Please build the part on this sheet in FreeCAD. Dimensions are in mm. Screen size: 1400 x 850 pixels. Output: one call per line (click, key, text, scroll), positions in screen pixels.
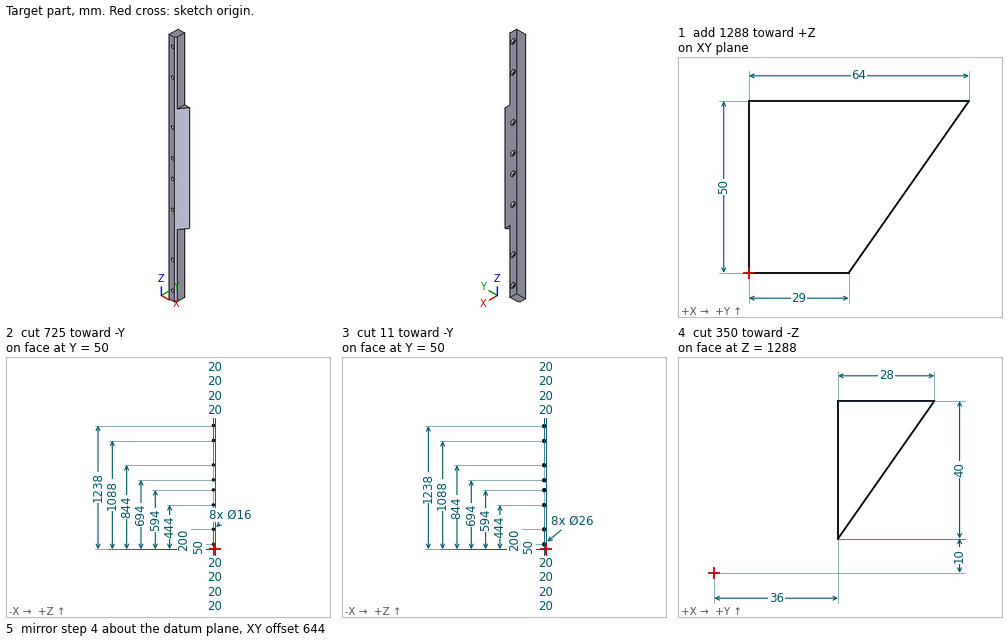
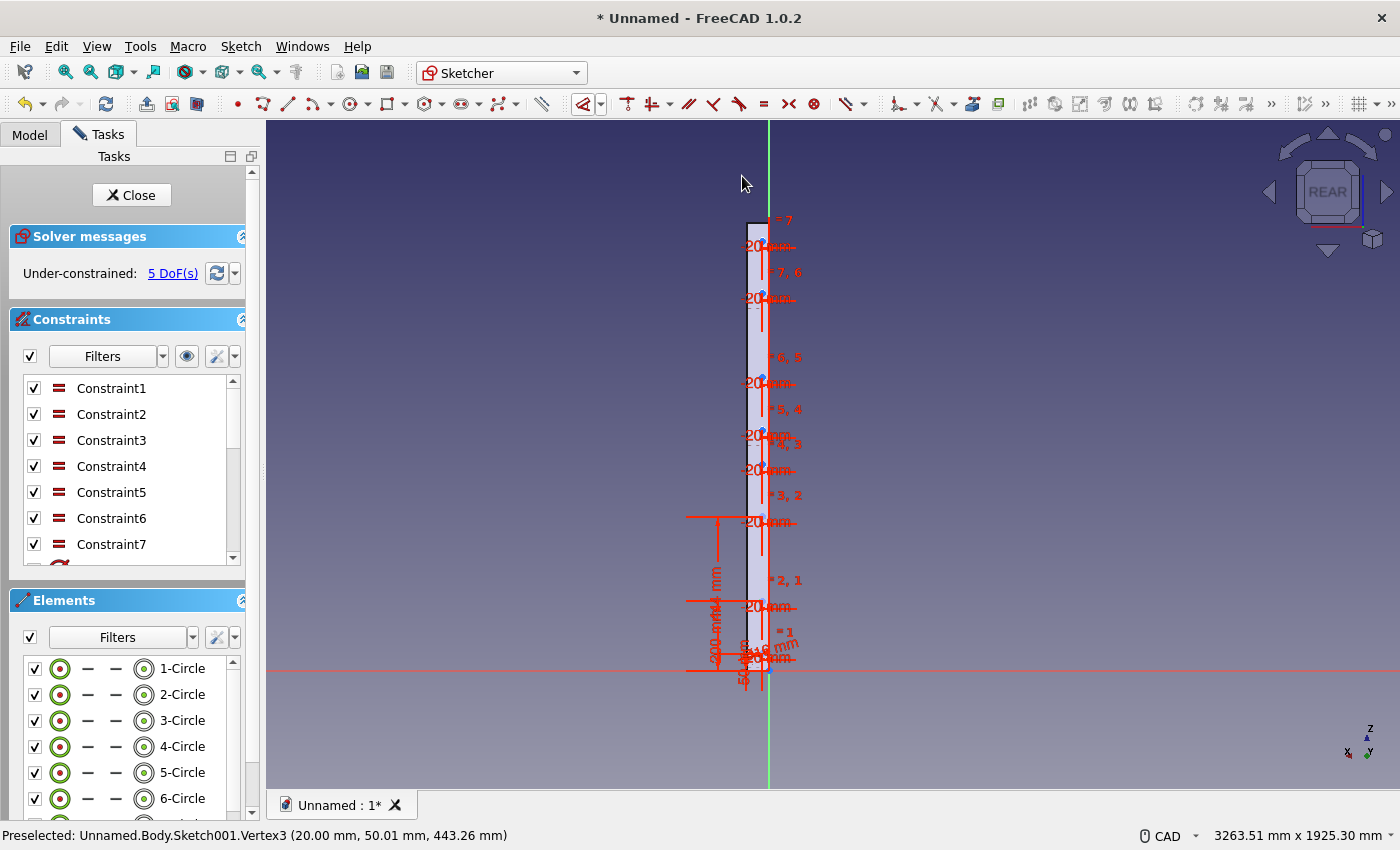
click(762, 465)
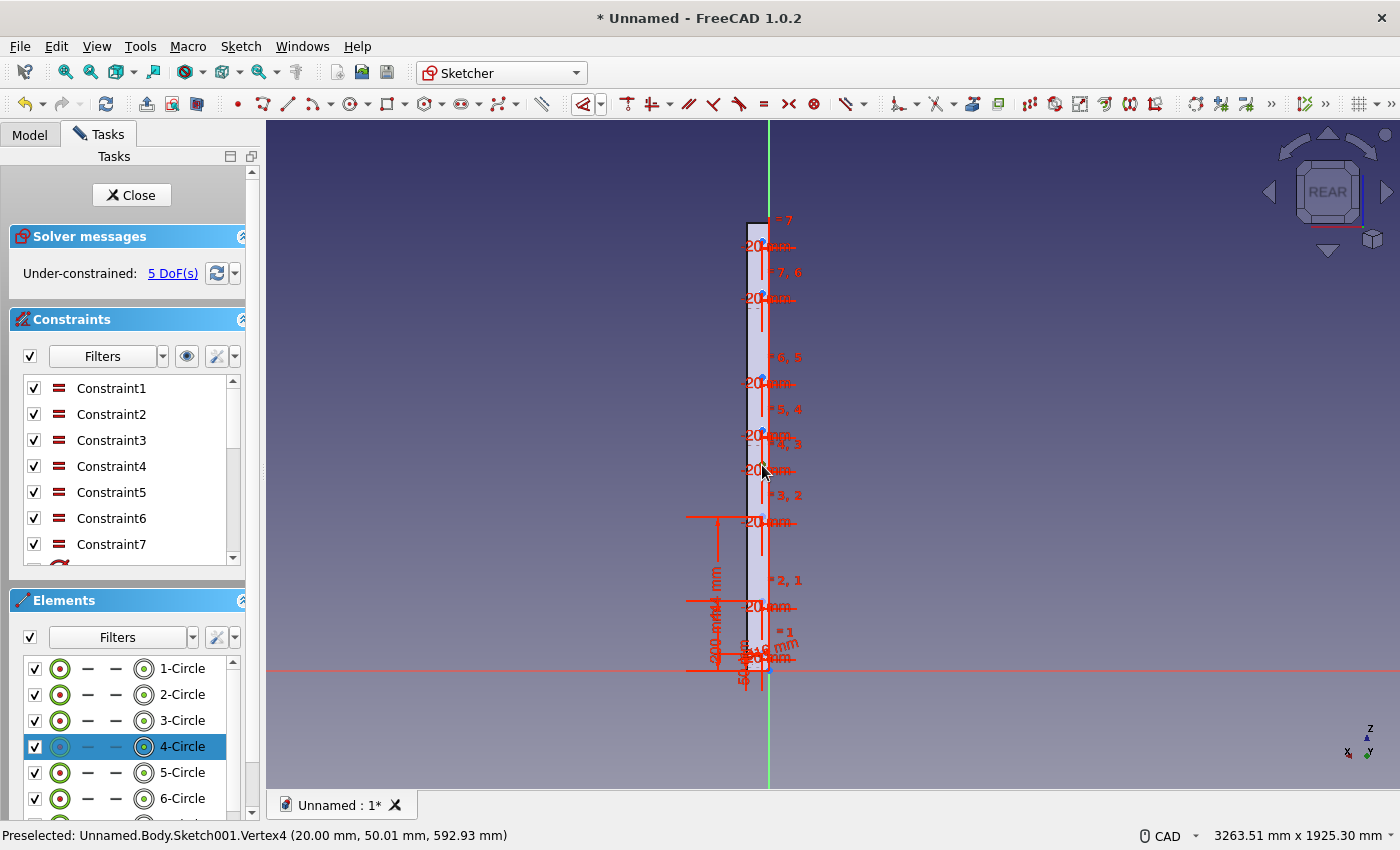
key(i)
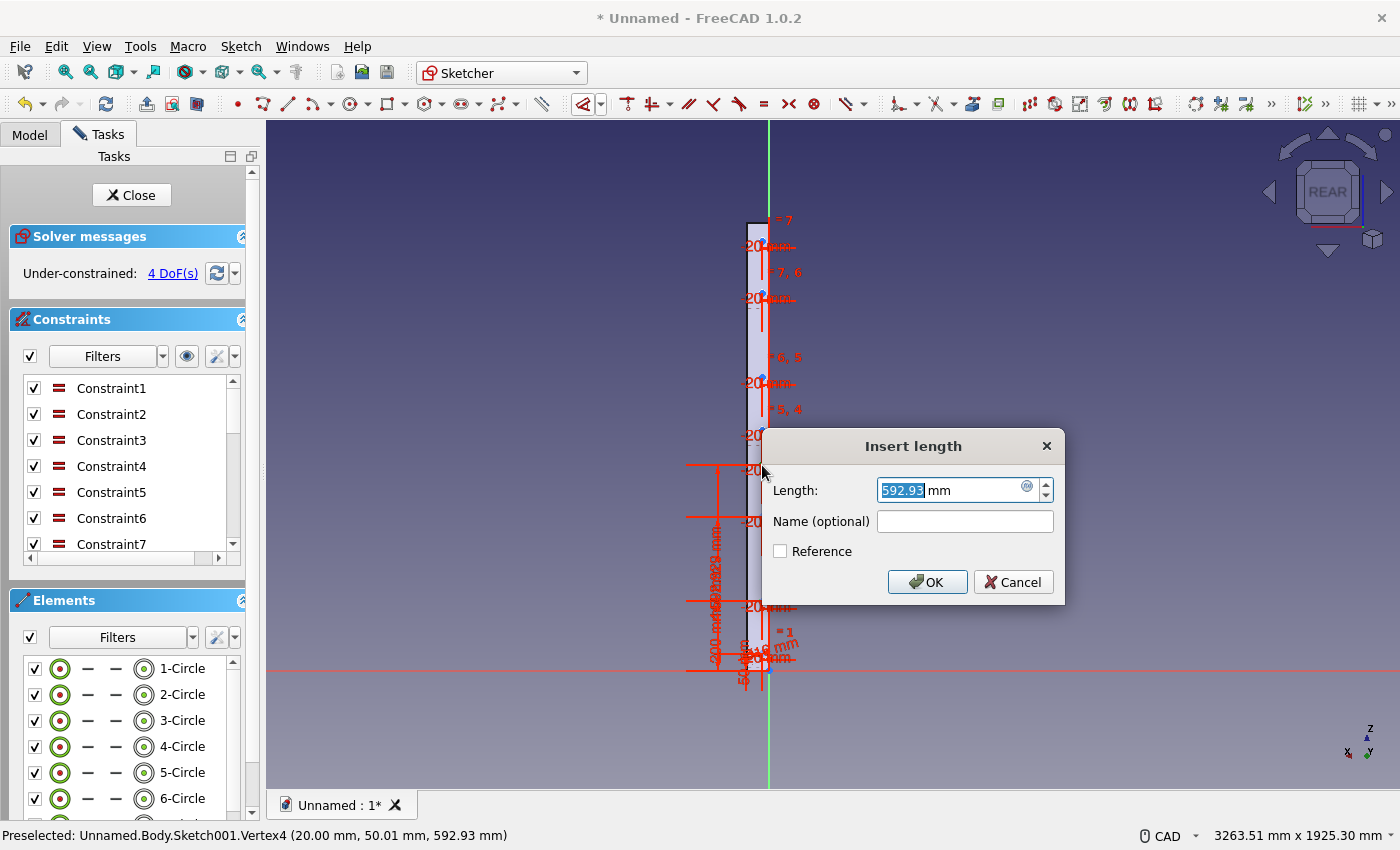
text(594)
key(Return)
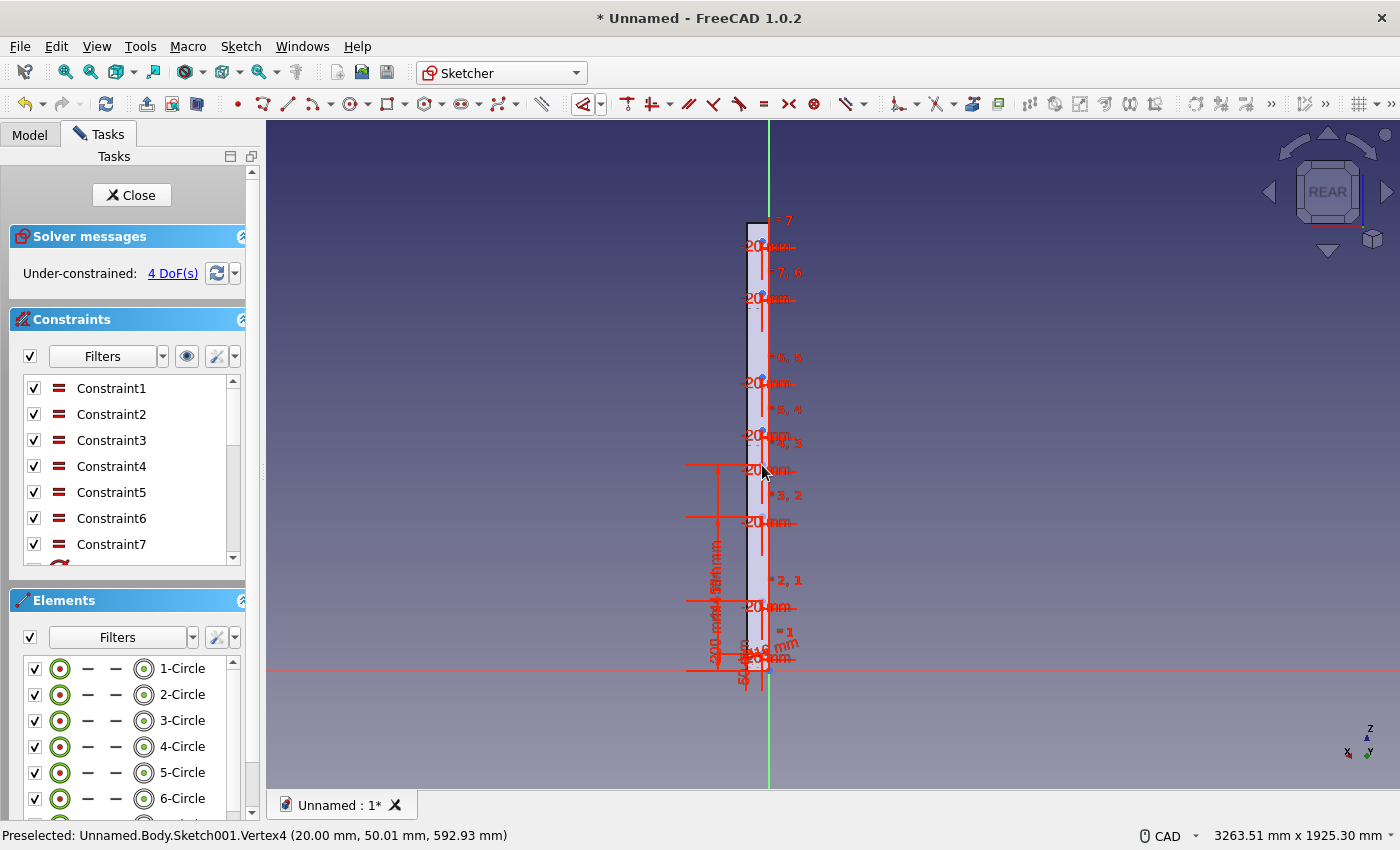
click(762, 430)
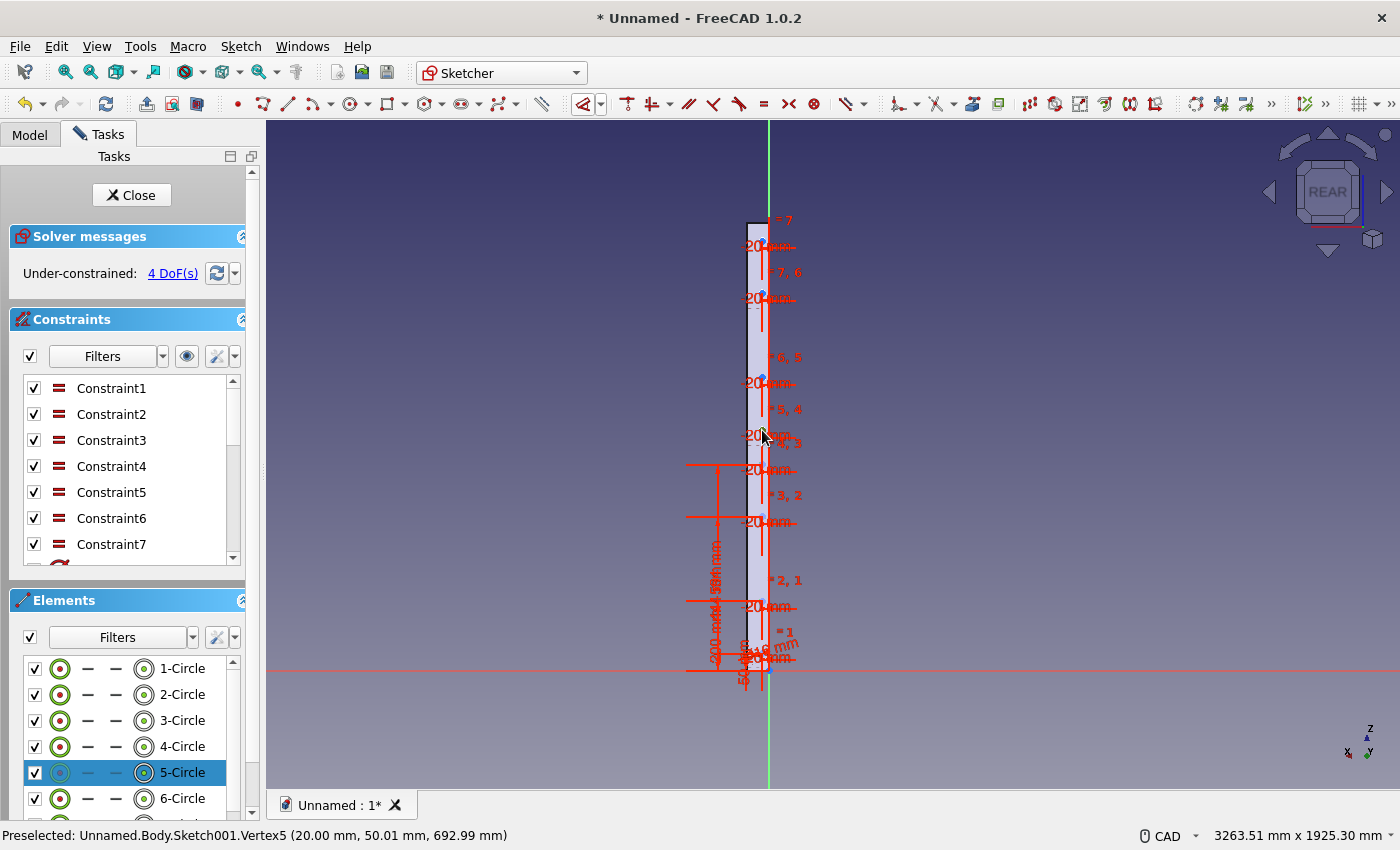
key(i)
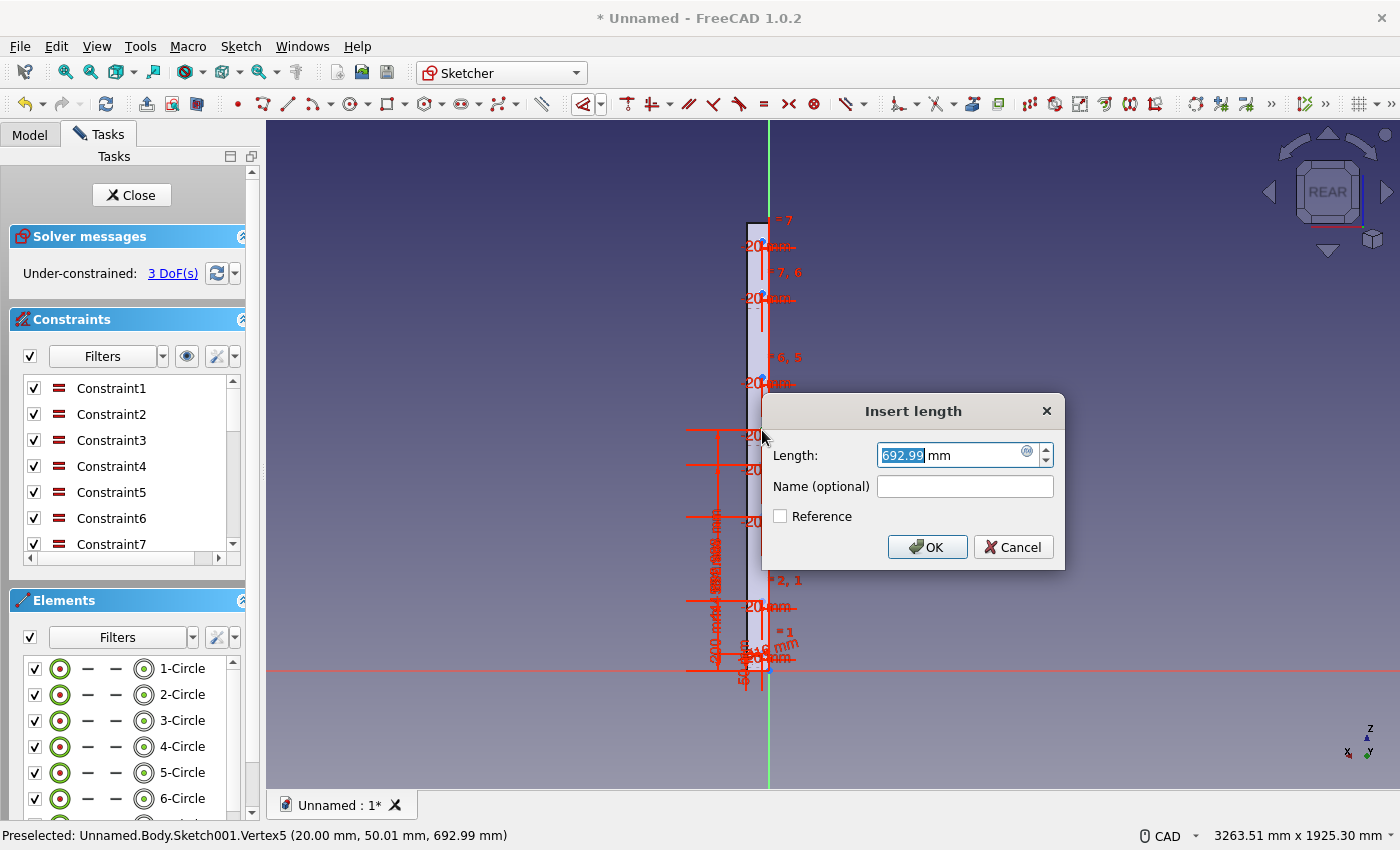
text(694)
key(Return)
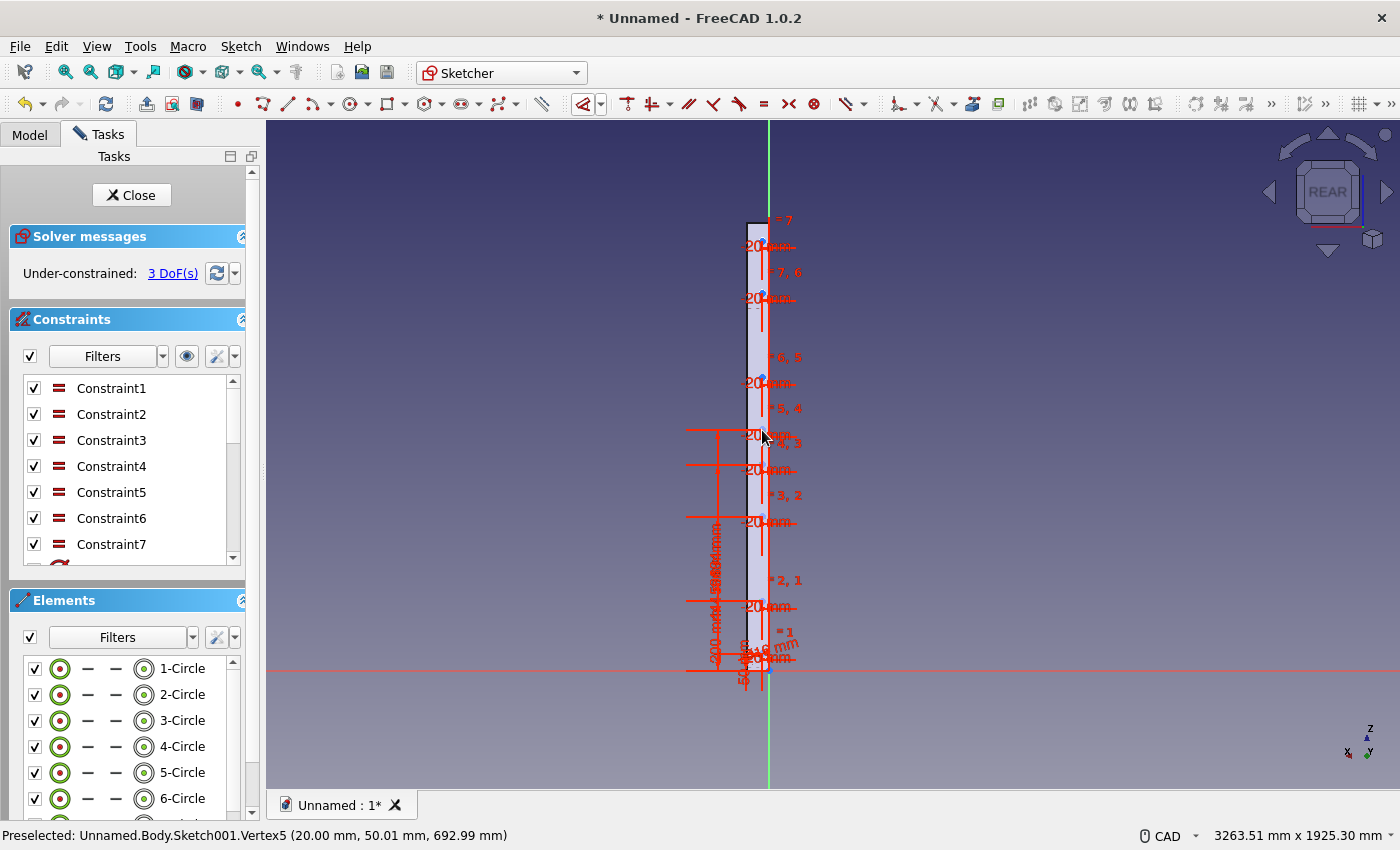
click(762, 378)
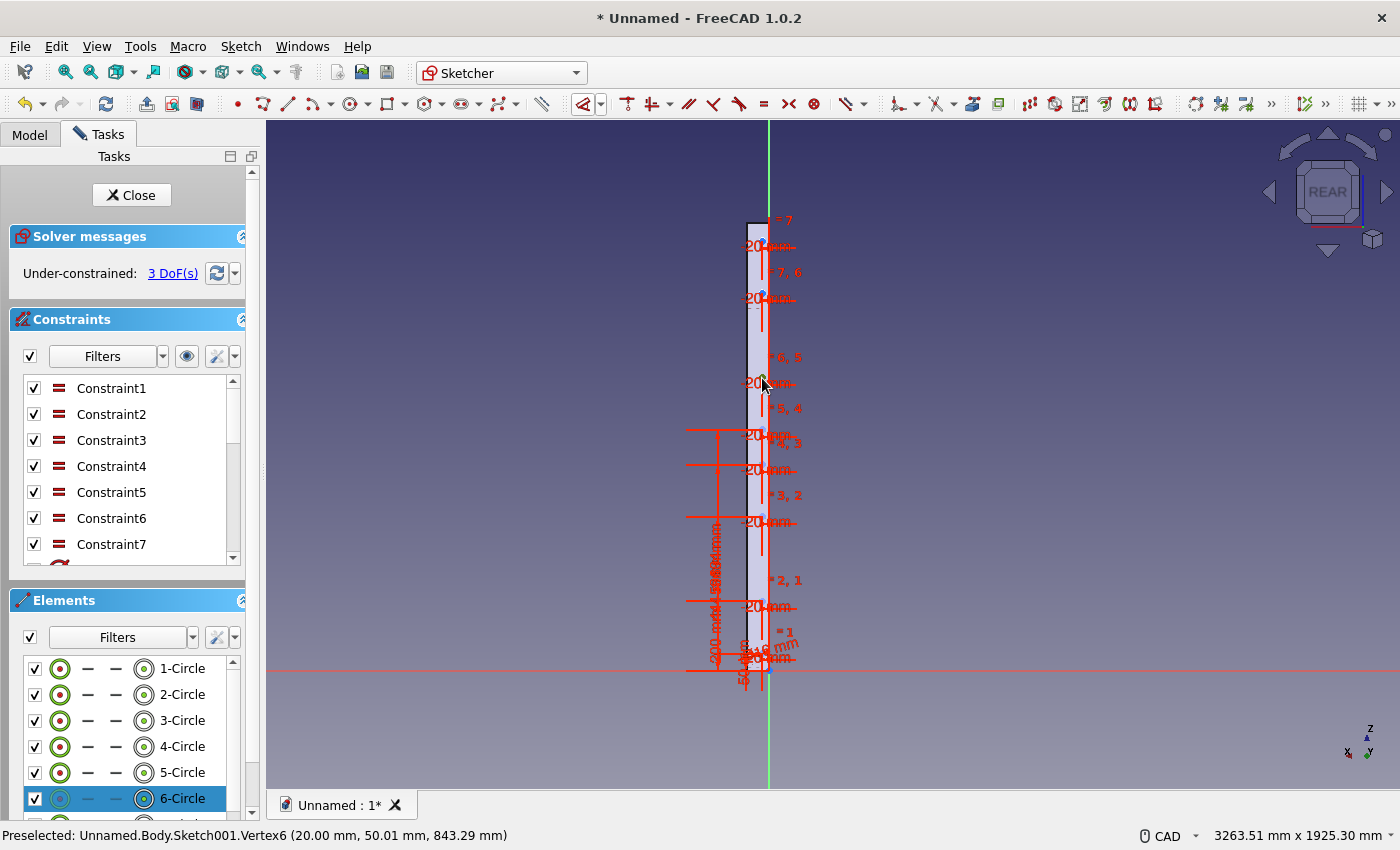
click(600, 104)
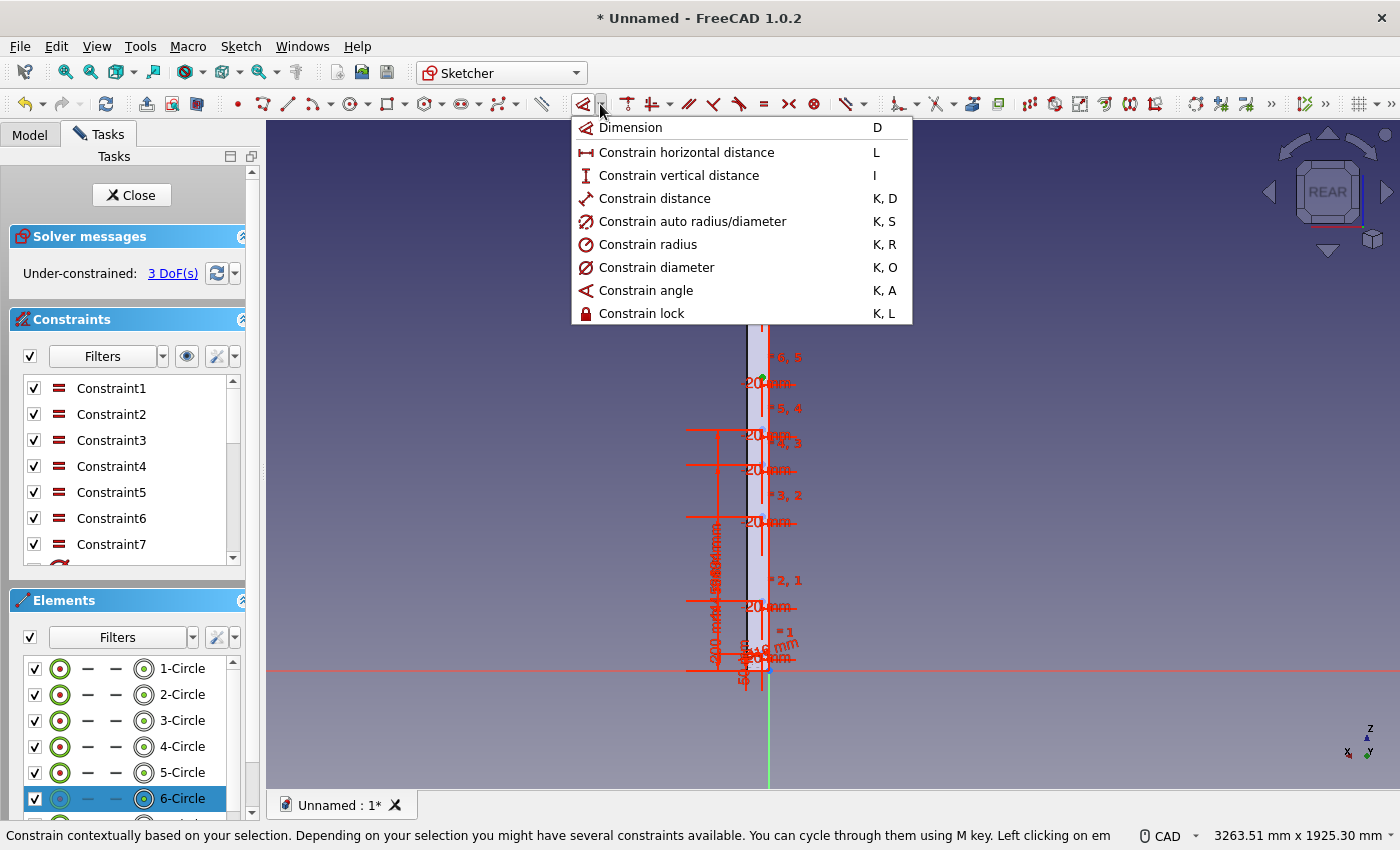
click(742, 176)